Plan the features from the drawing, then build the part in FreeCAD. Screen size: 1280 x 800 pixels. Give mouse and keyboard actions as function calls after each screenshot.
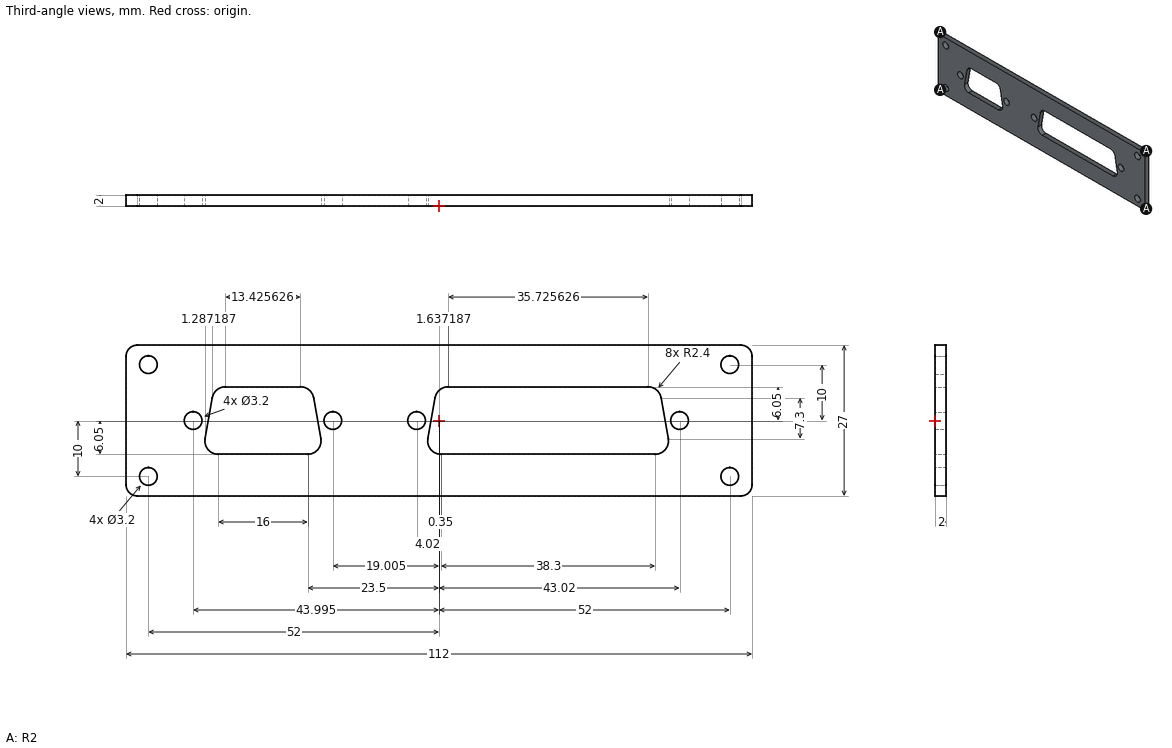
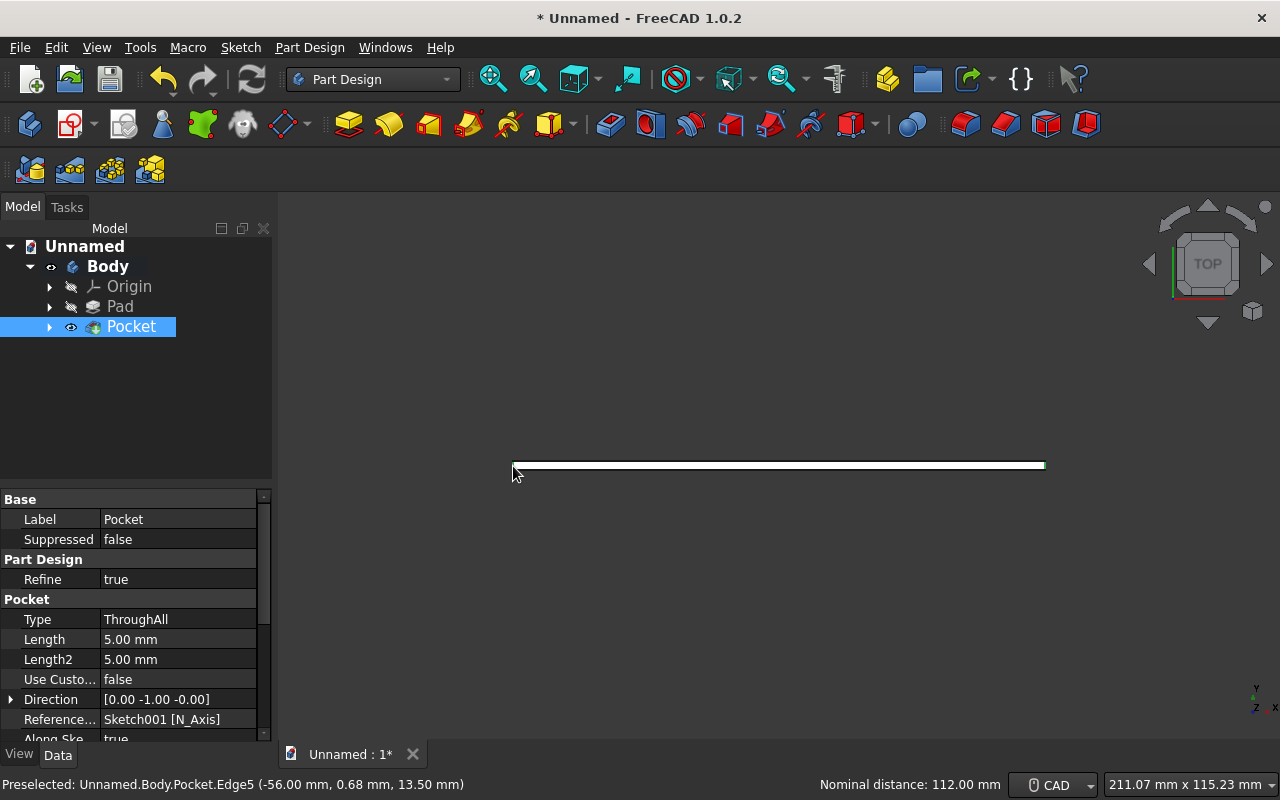
scroll(513, 464, up, 8)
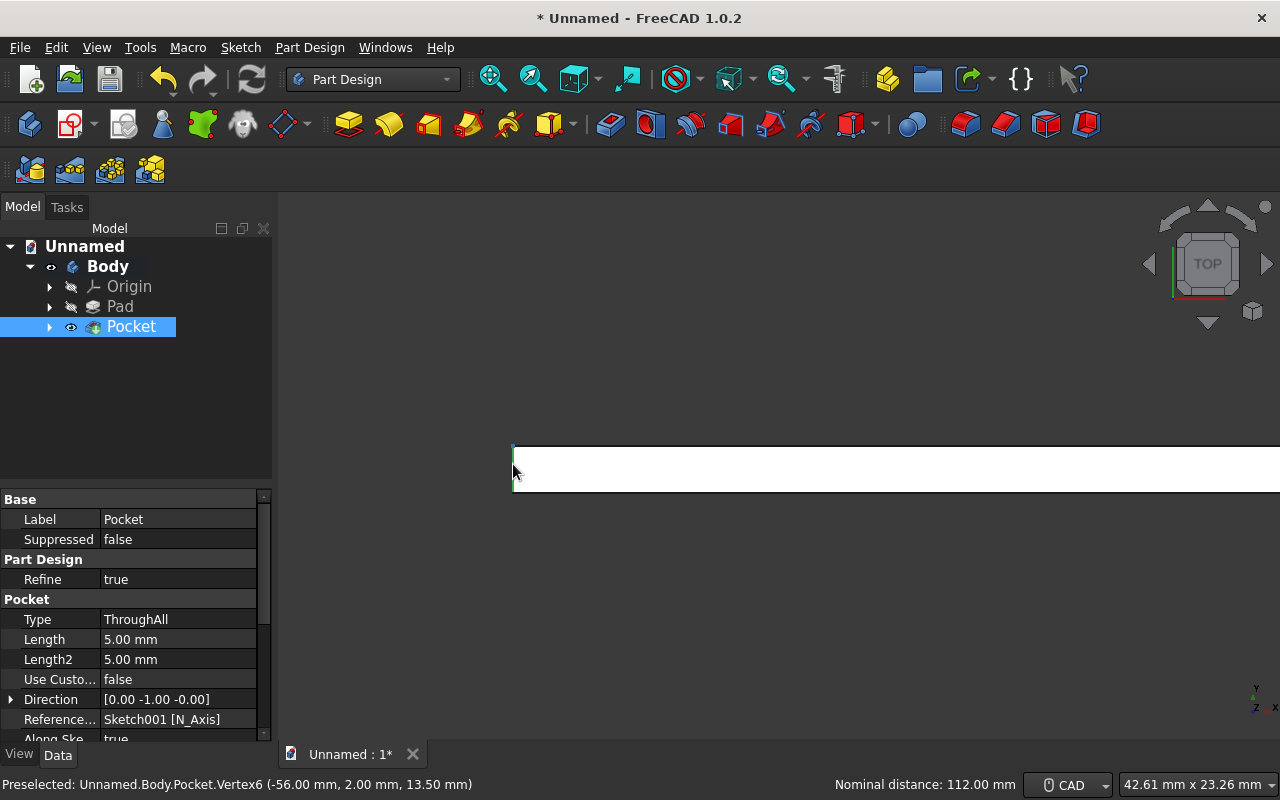
click(494, 80)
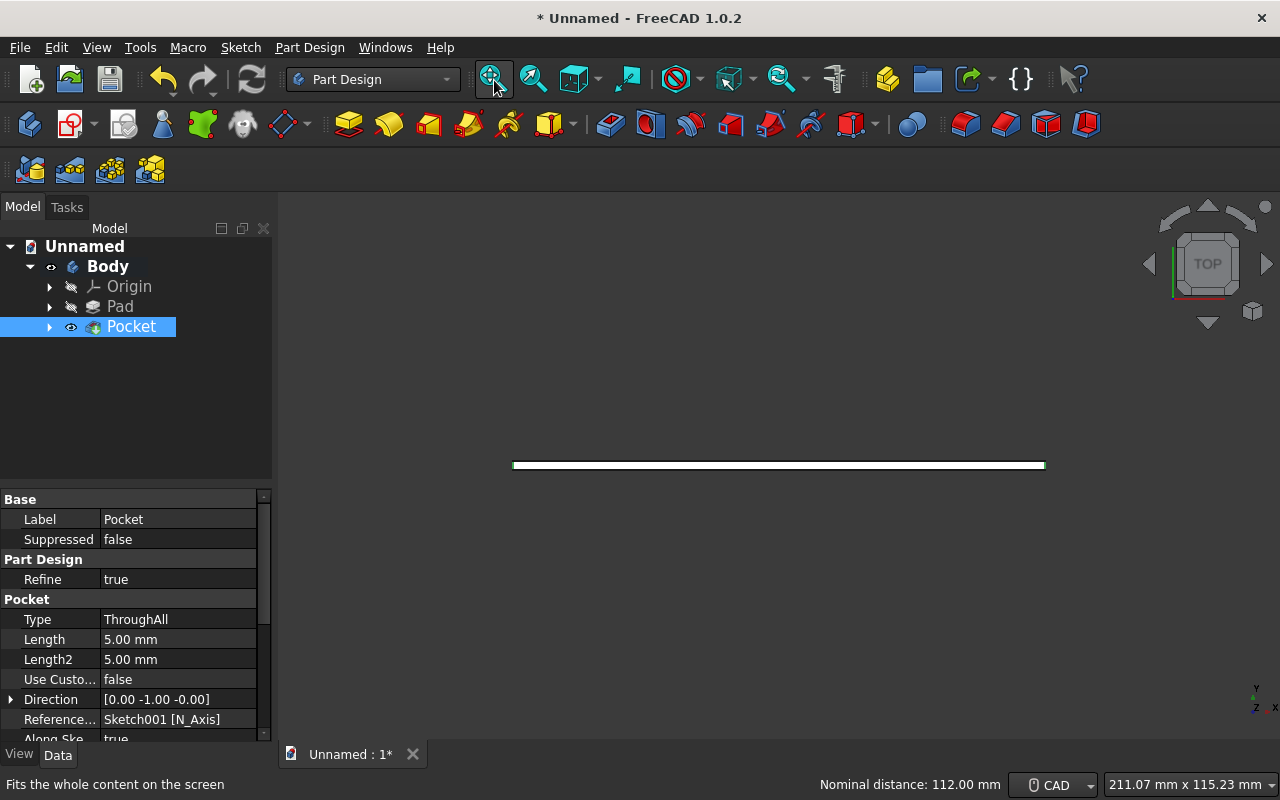
key(1)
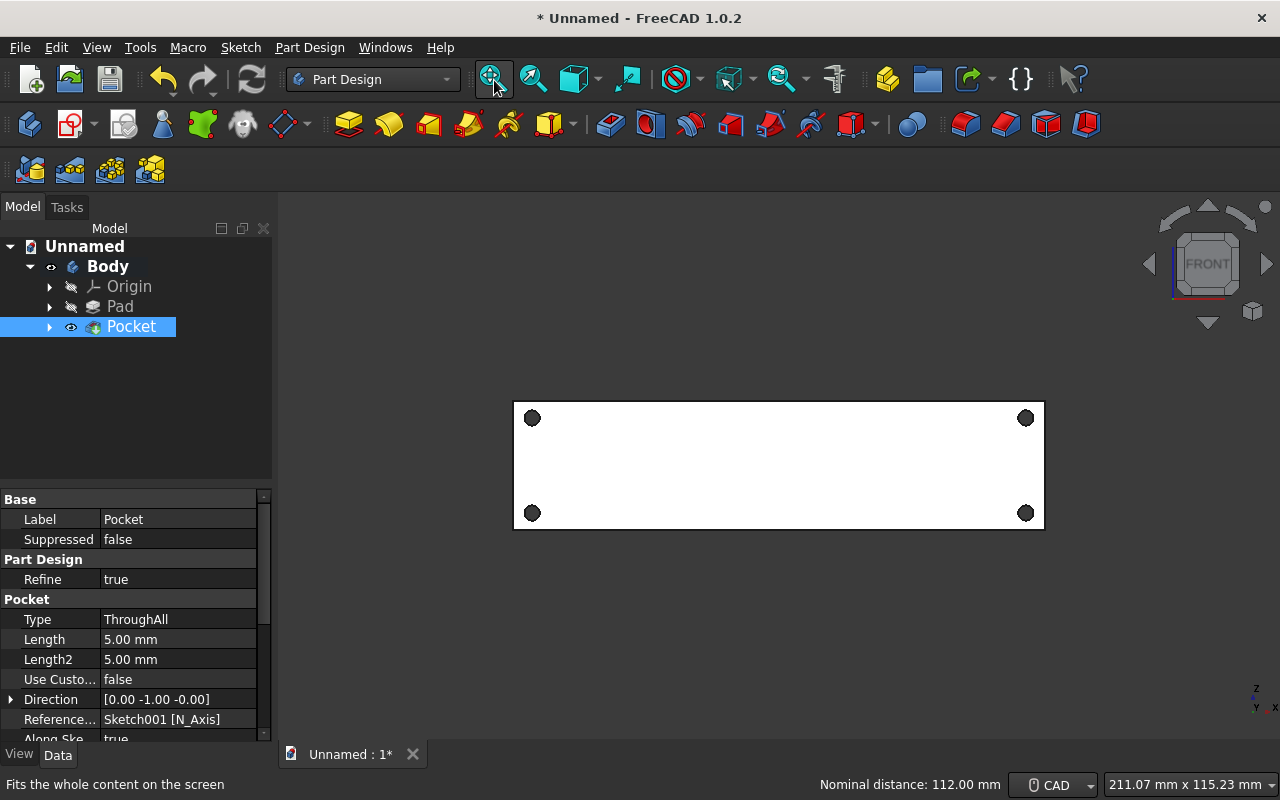
scroll(513, 529, up, 8)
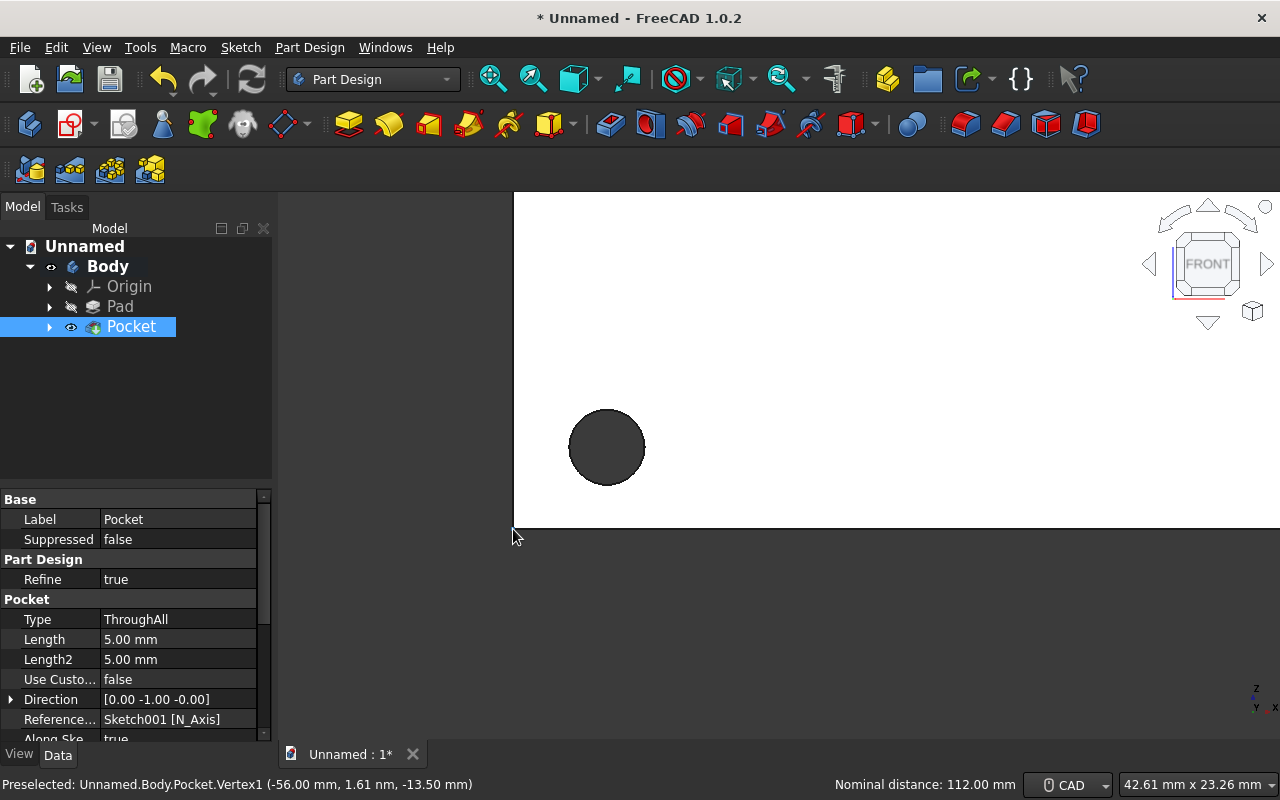
click(494, 80)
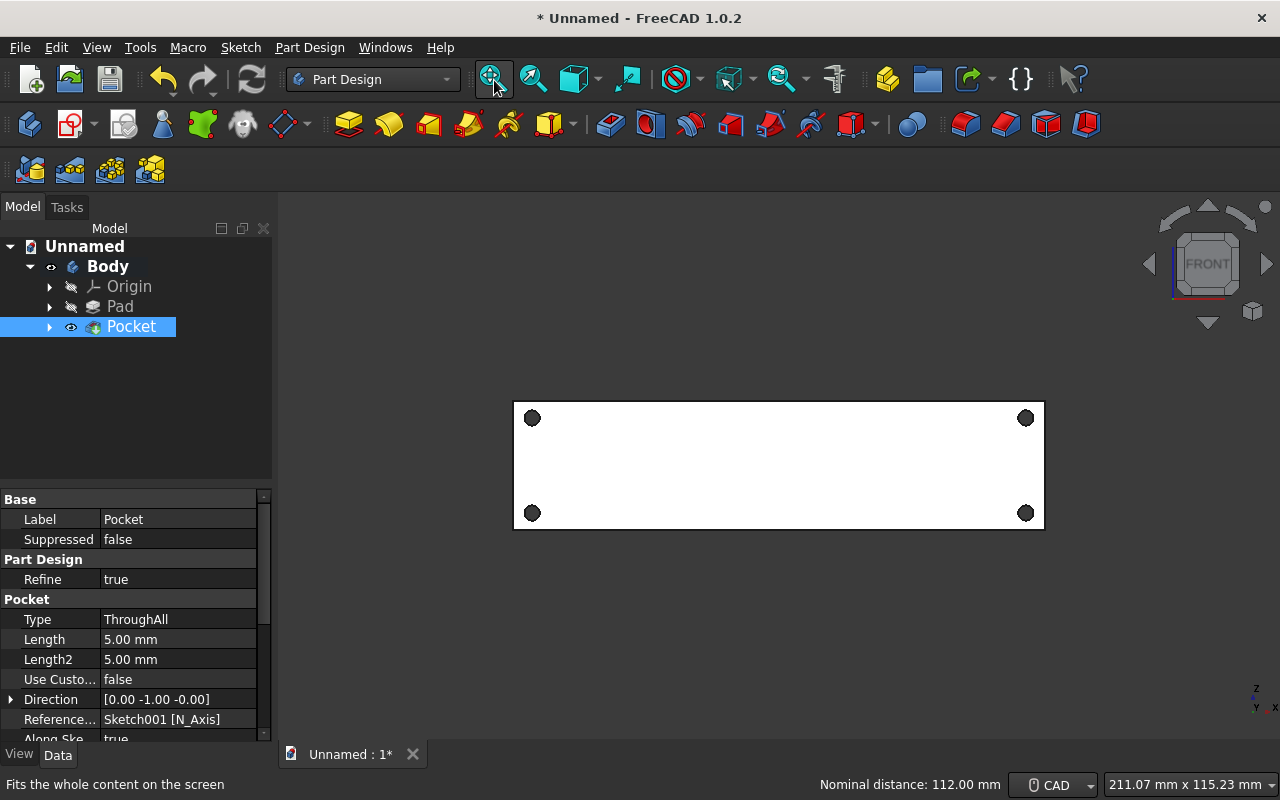
key(3)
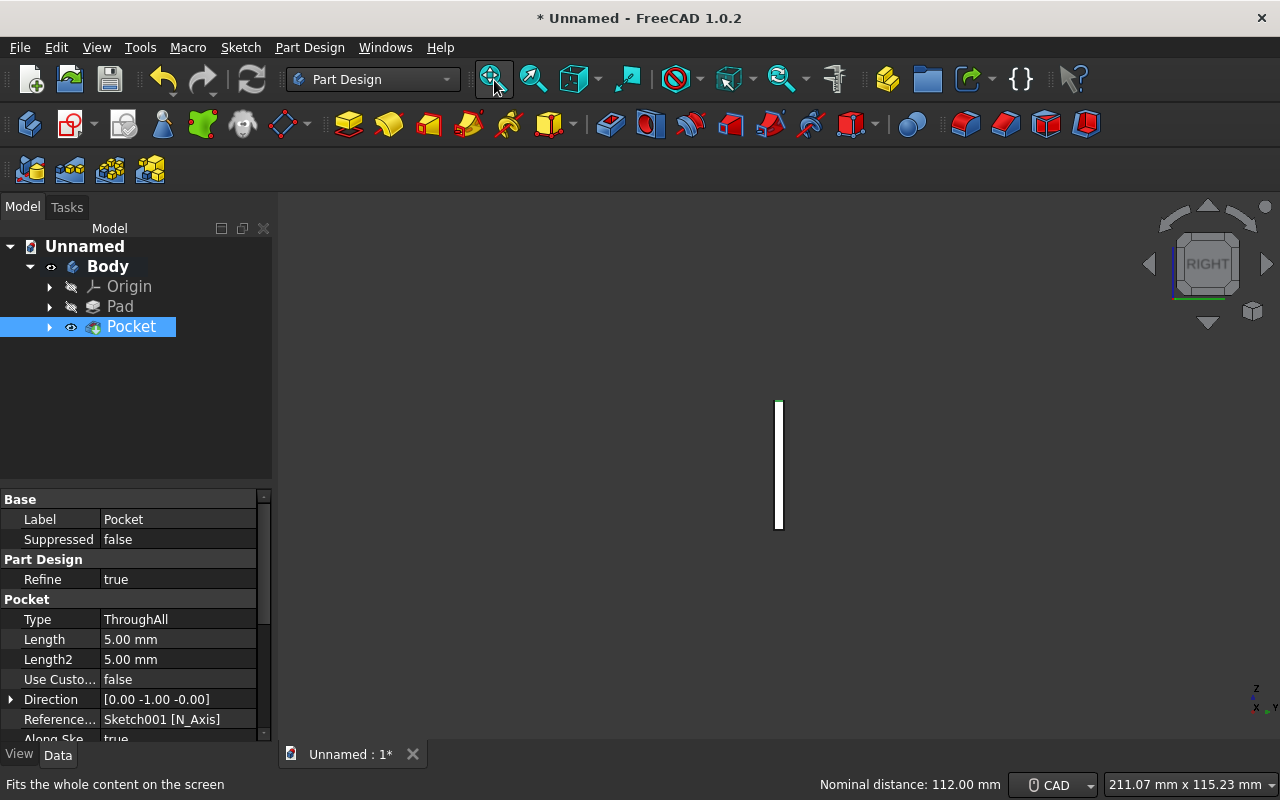
key(v)
key(f)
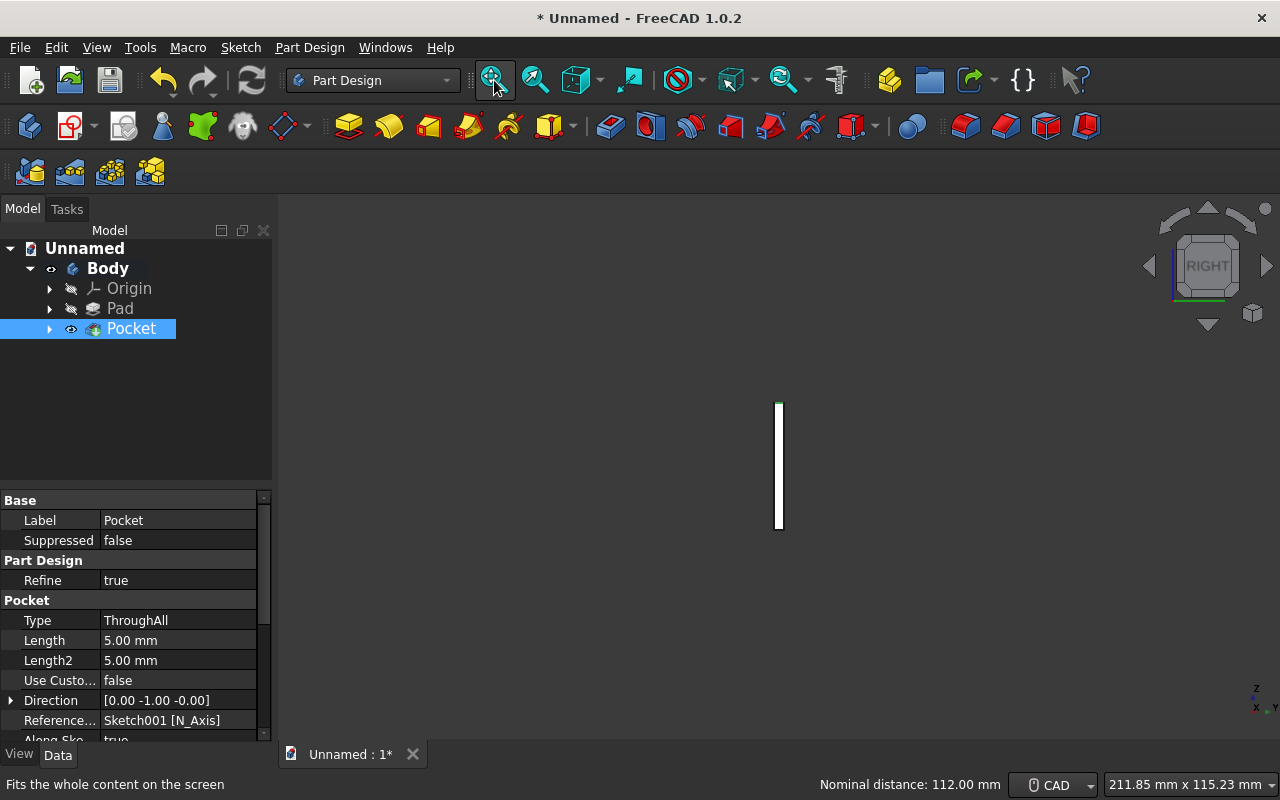
scroll(779, 529, up, 8)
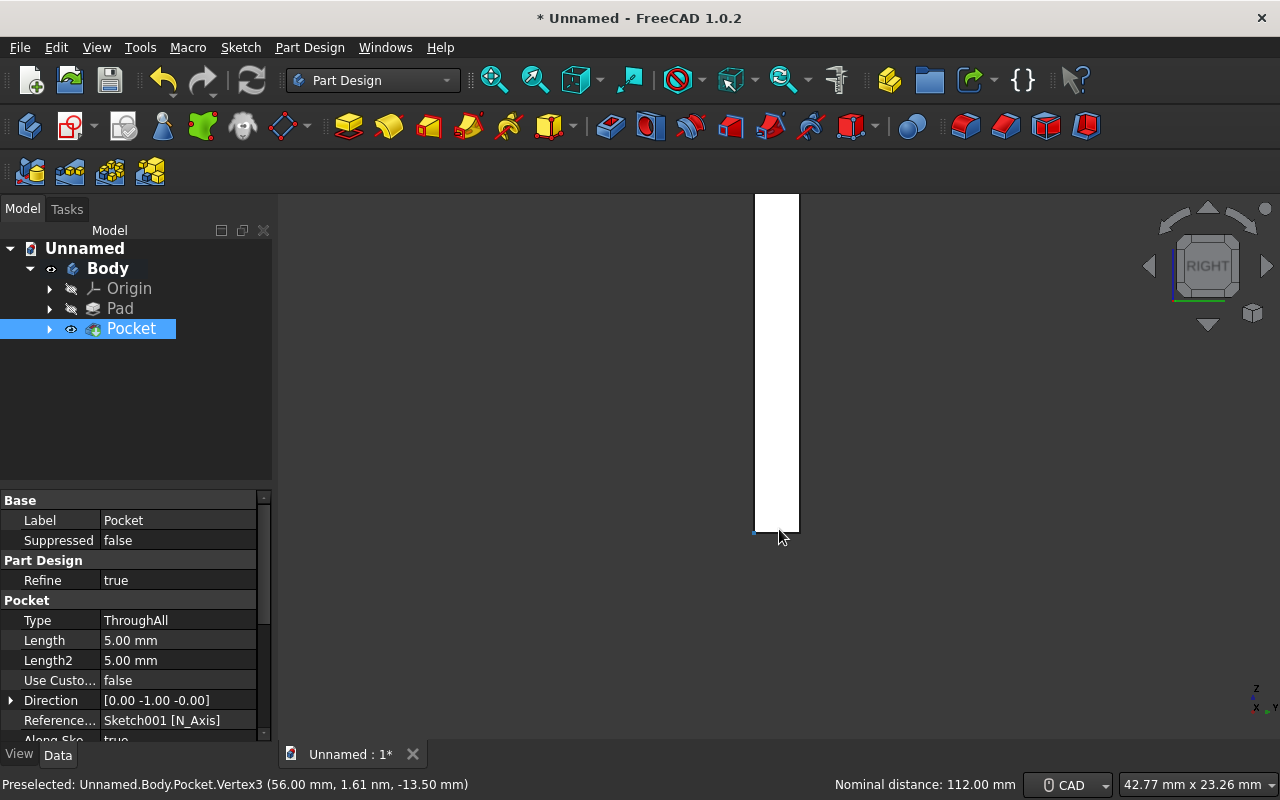
click(777, 532, ctrl)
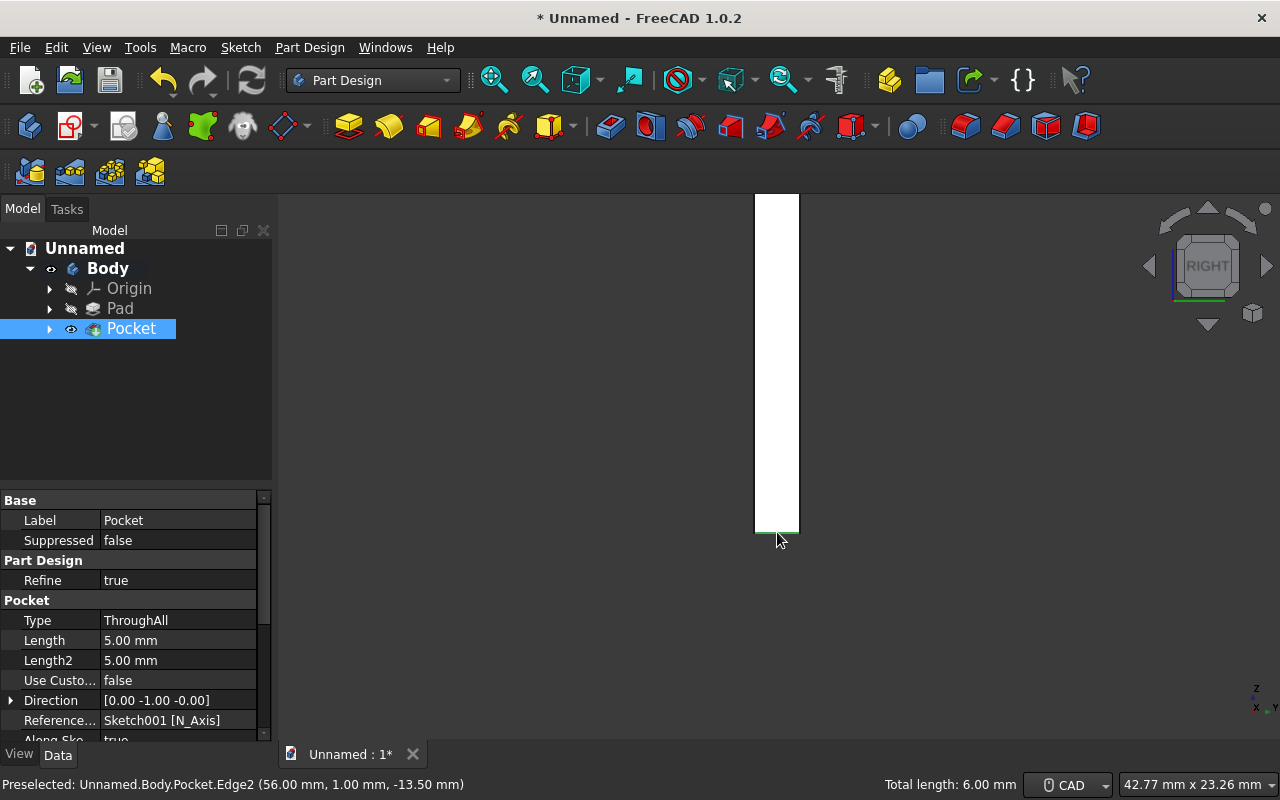
click(496, 80)